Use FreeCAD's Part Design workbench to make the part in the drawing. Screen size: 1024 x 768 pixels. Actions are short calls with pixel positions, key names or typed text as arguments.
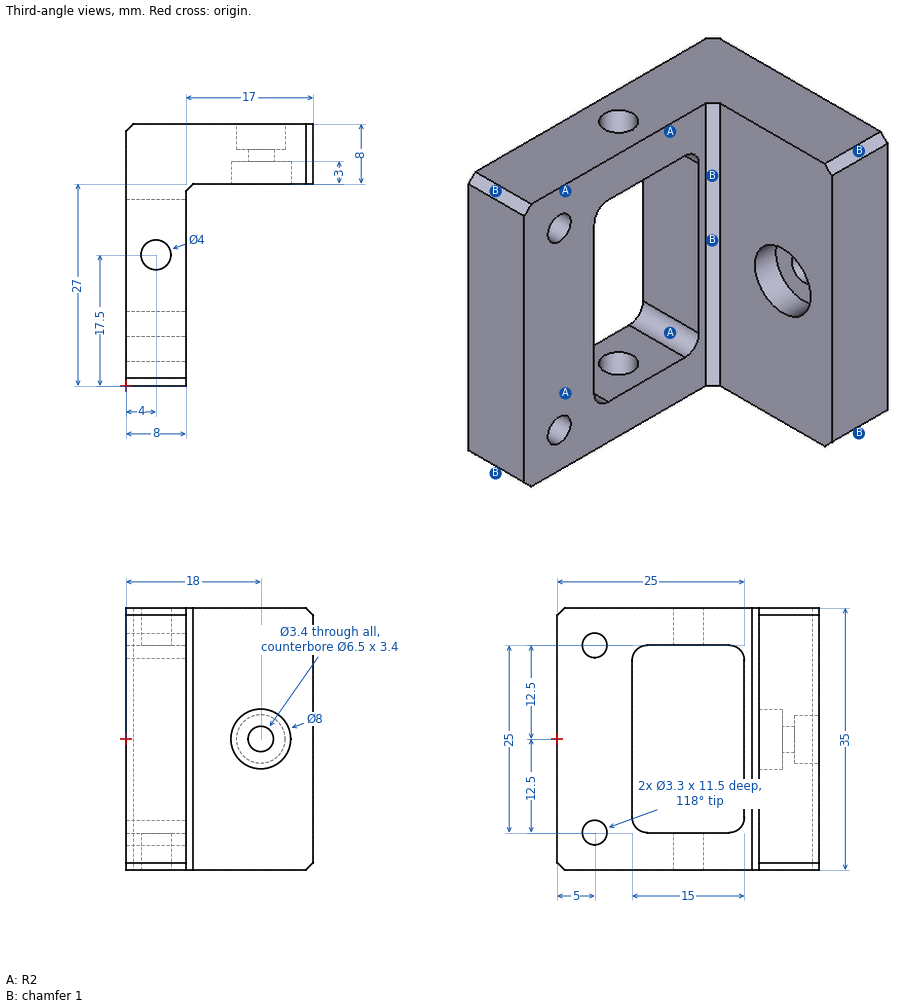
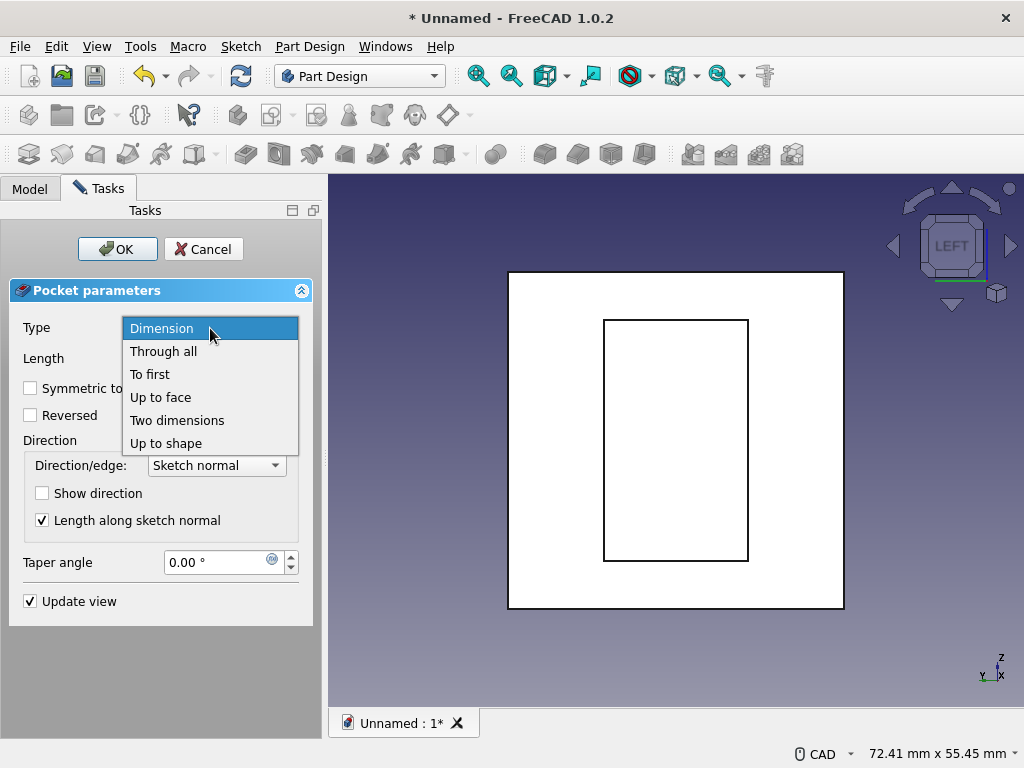
click(208, 352)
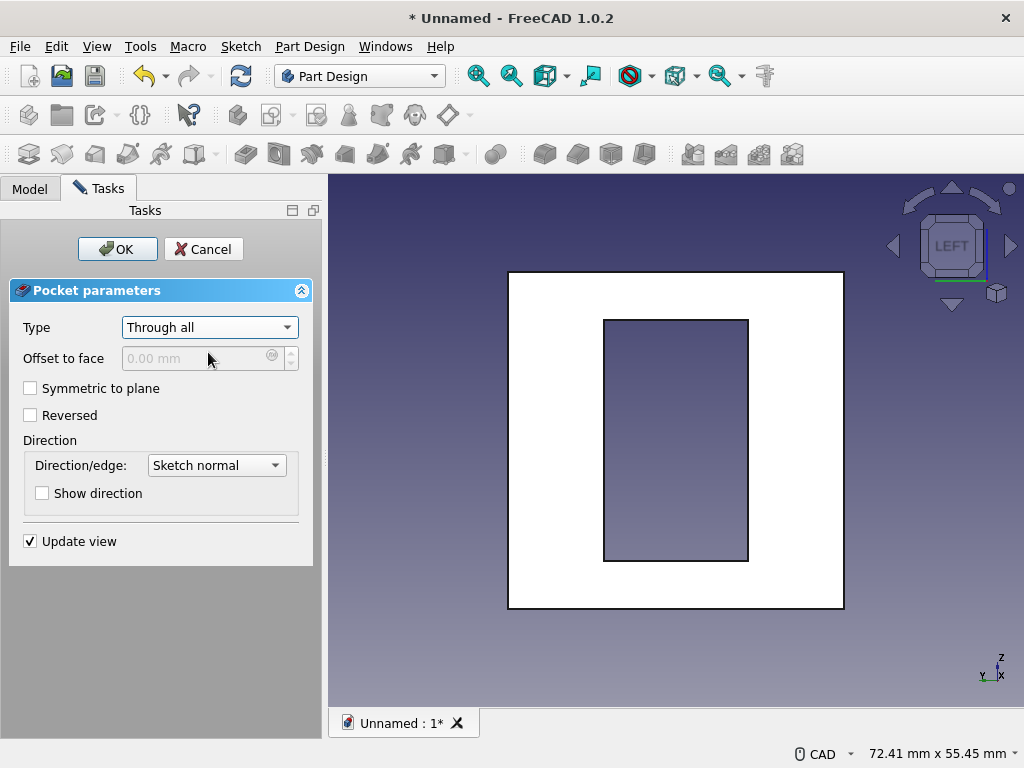
click(118, 249)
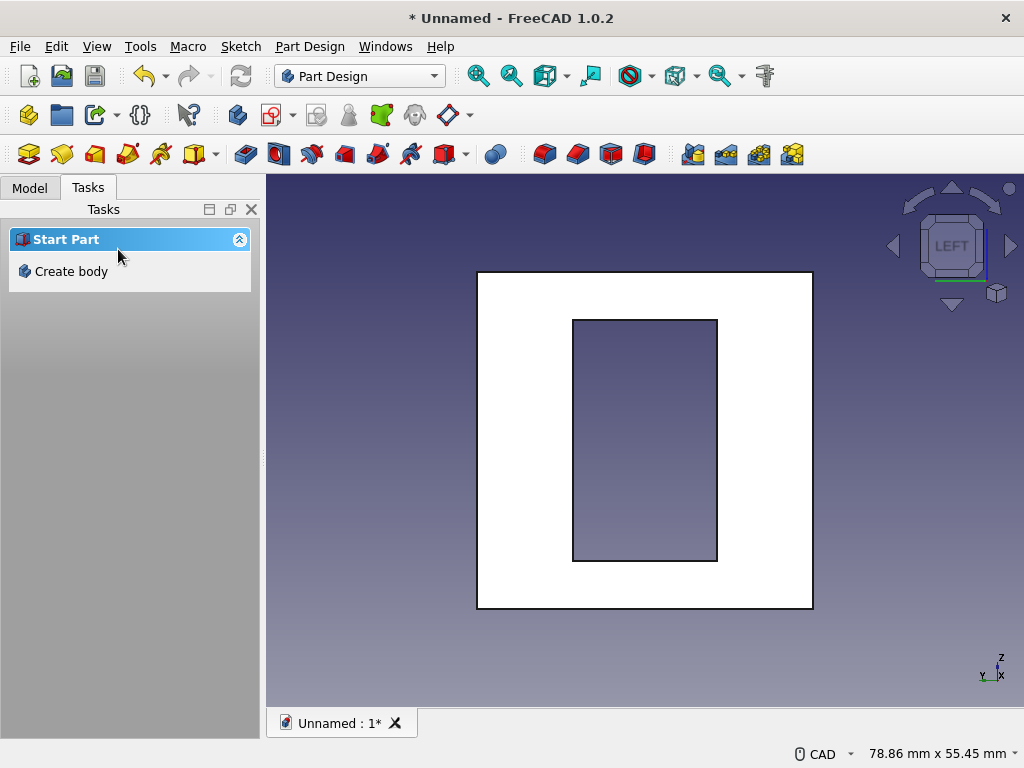
click(270, 116)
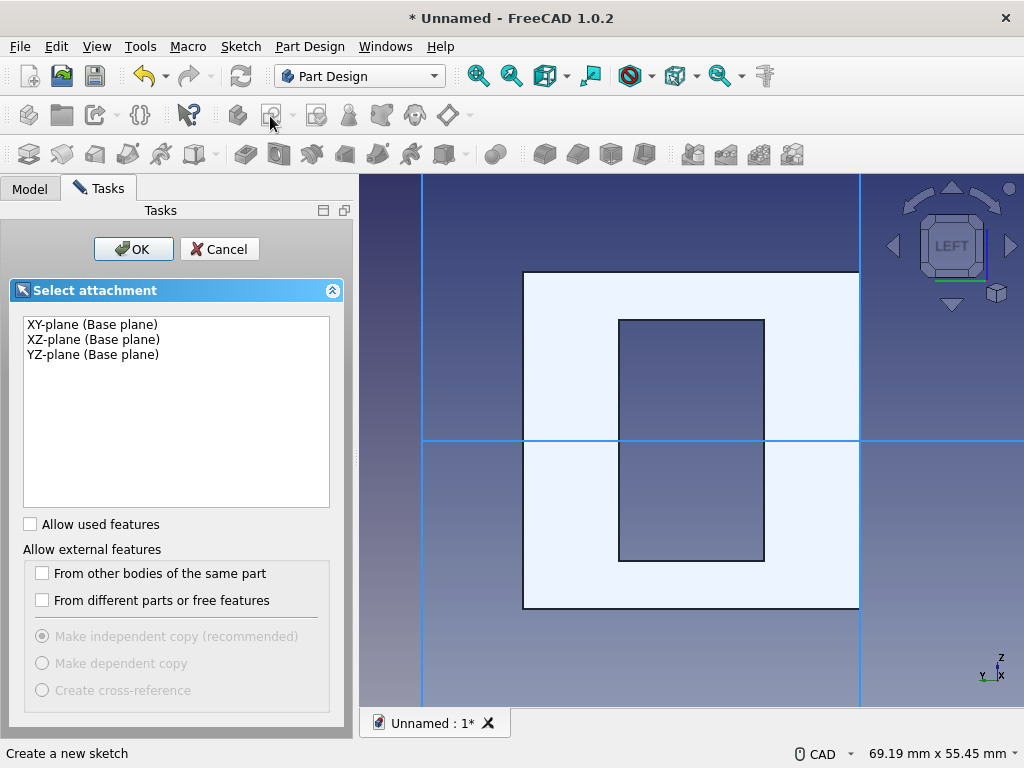
click(84, 354)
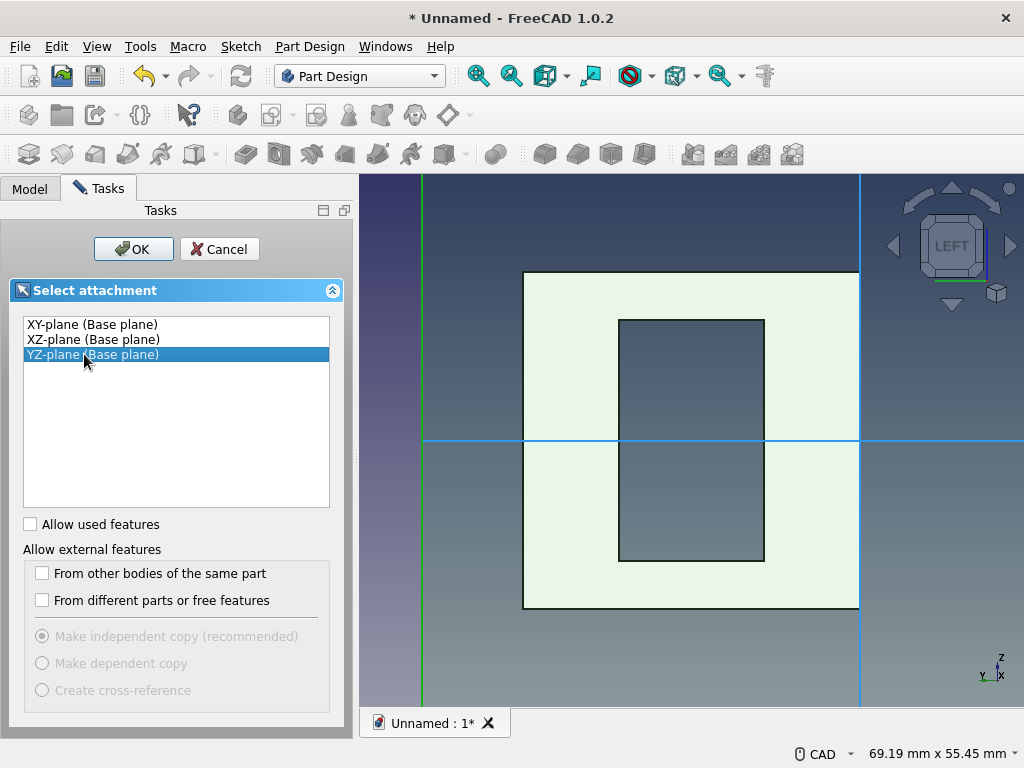
click(134, 249)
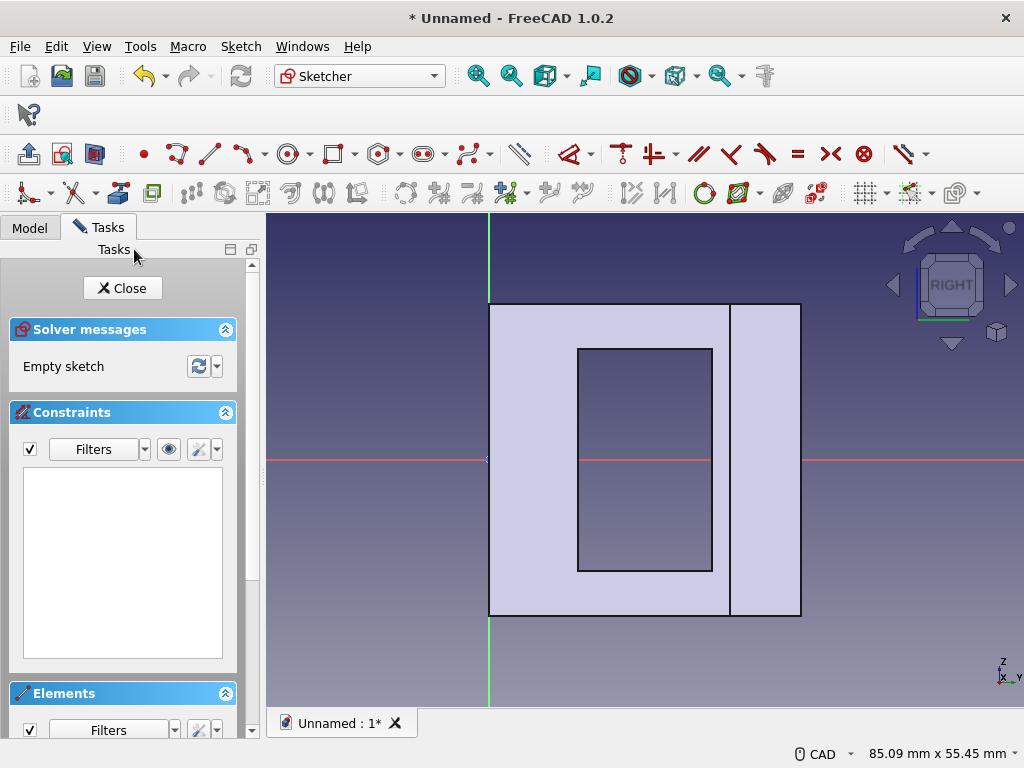
key(q)
key(s)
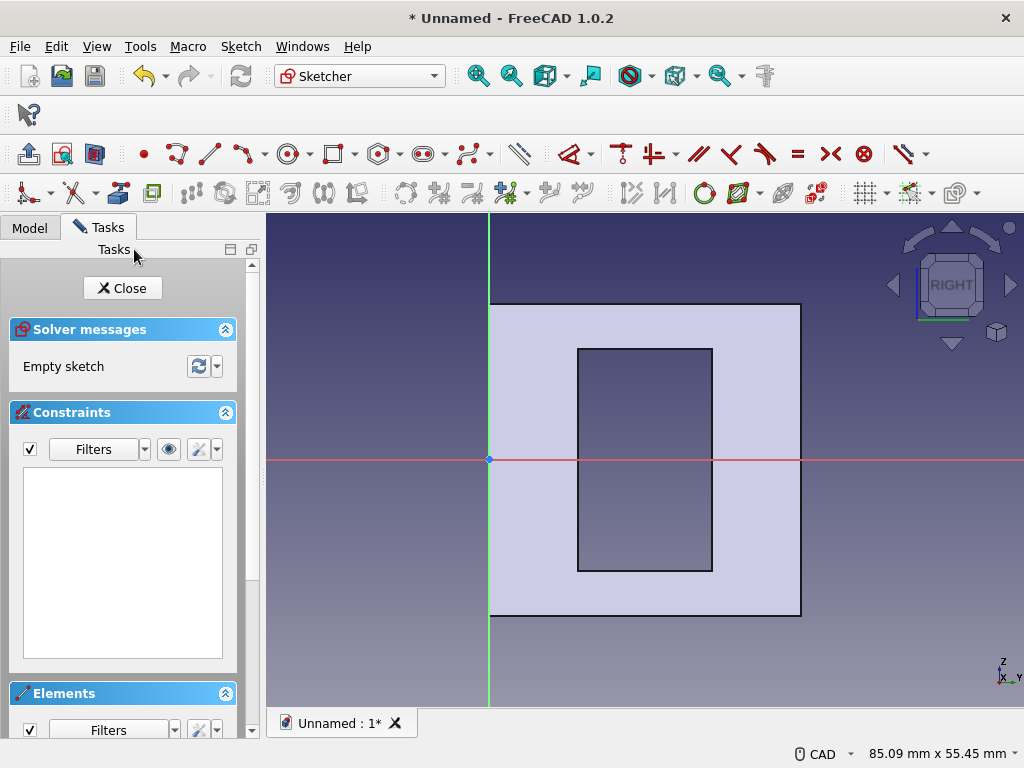
key(g)
key(c)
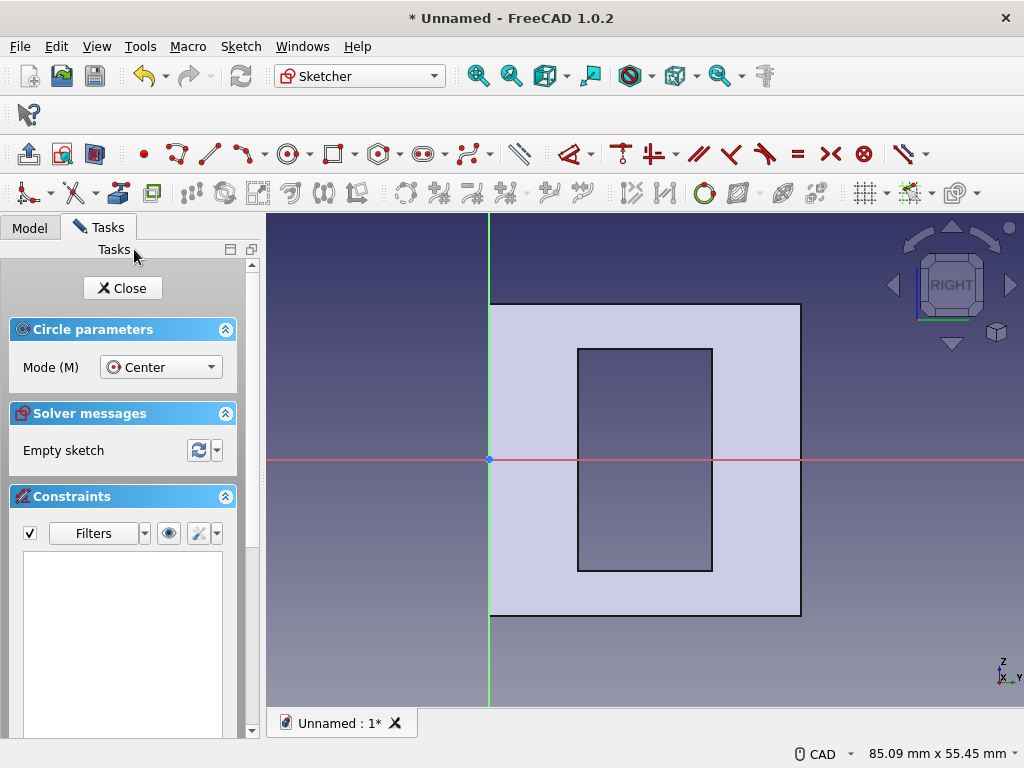
scroll(534, 571, up, 3)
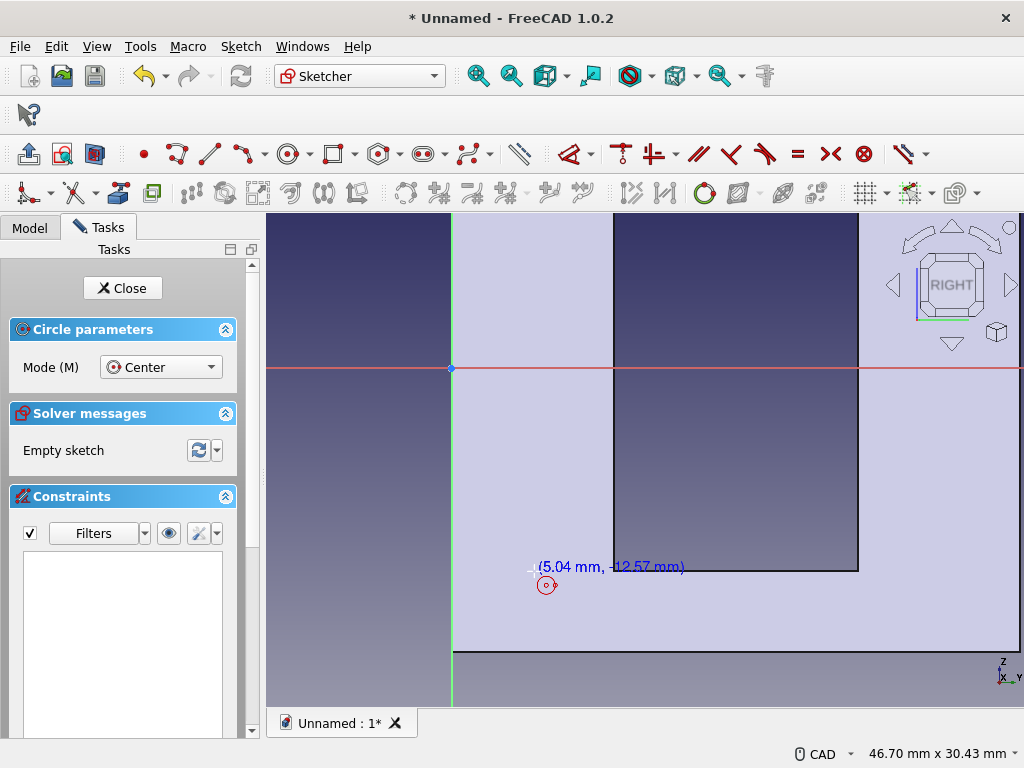
click(533, 571)
move(552, 552)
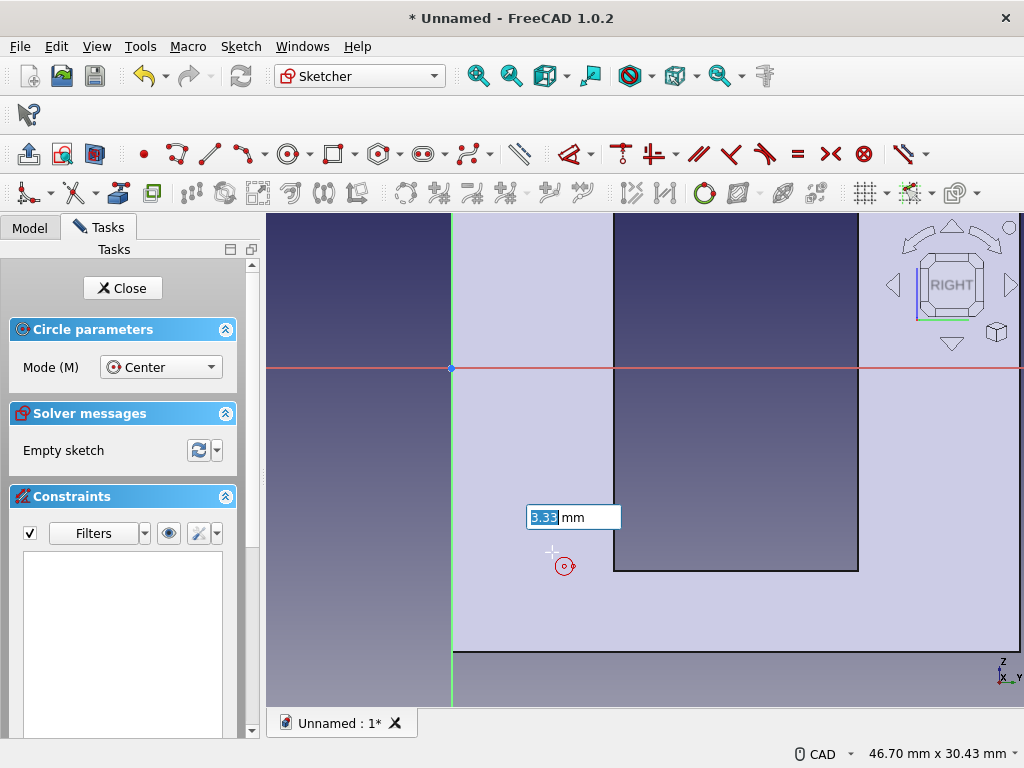
text(3.3)
key(Return)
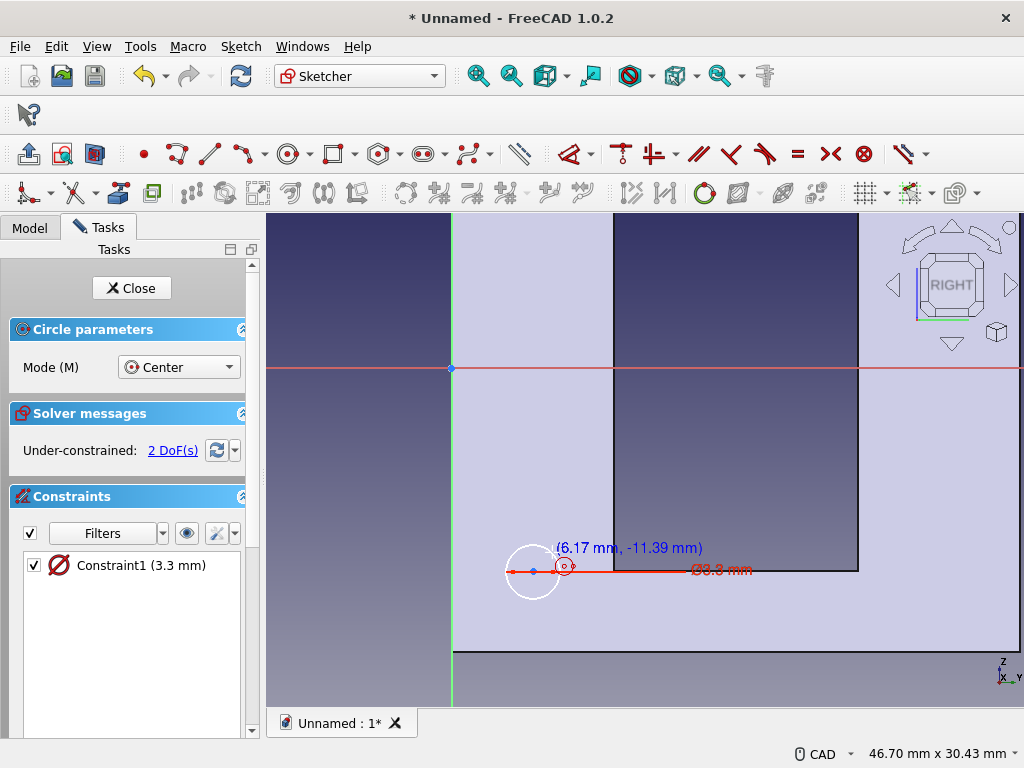
scroll(720, 647, down, 2)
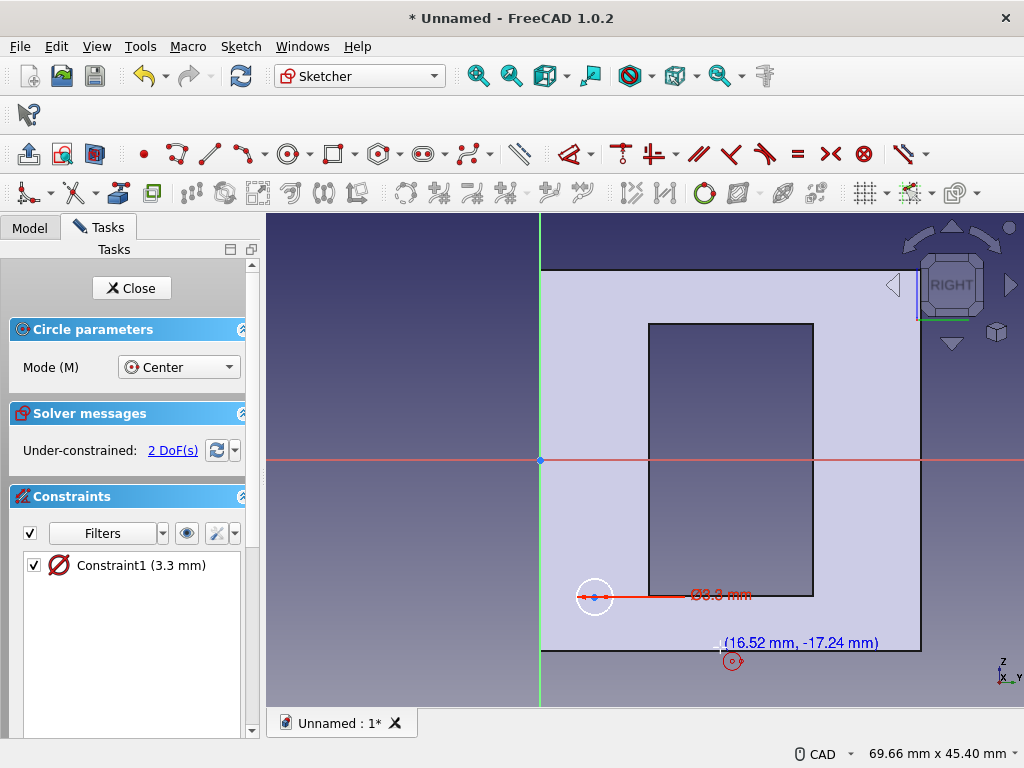
scroll(595, 324, up, 2)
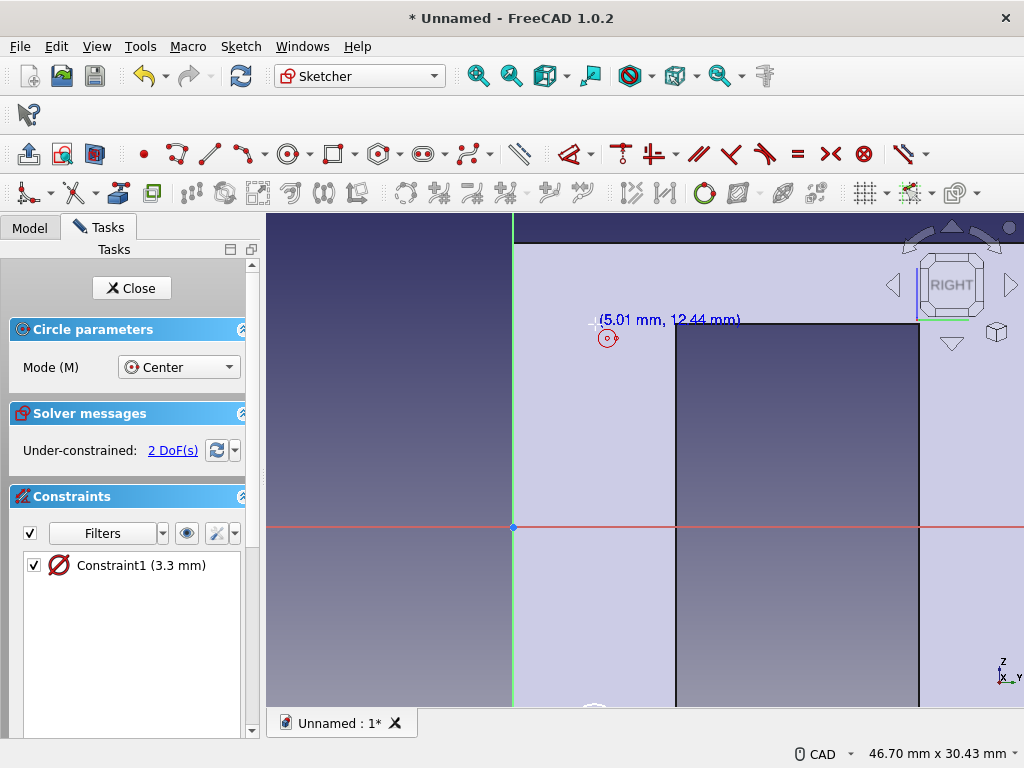
click(595, 324)
move(614, 305)